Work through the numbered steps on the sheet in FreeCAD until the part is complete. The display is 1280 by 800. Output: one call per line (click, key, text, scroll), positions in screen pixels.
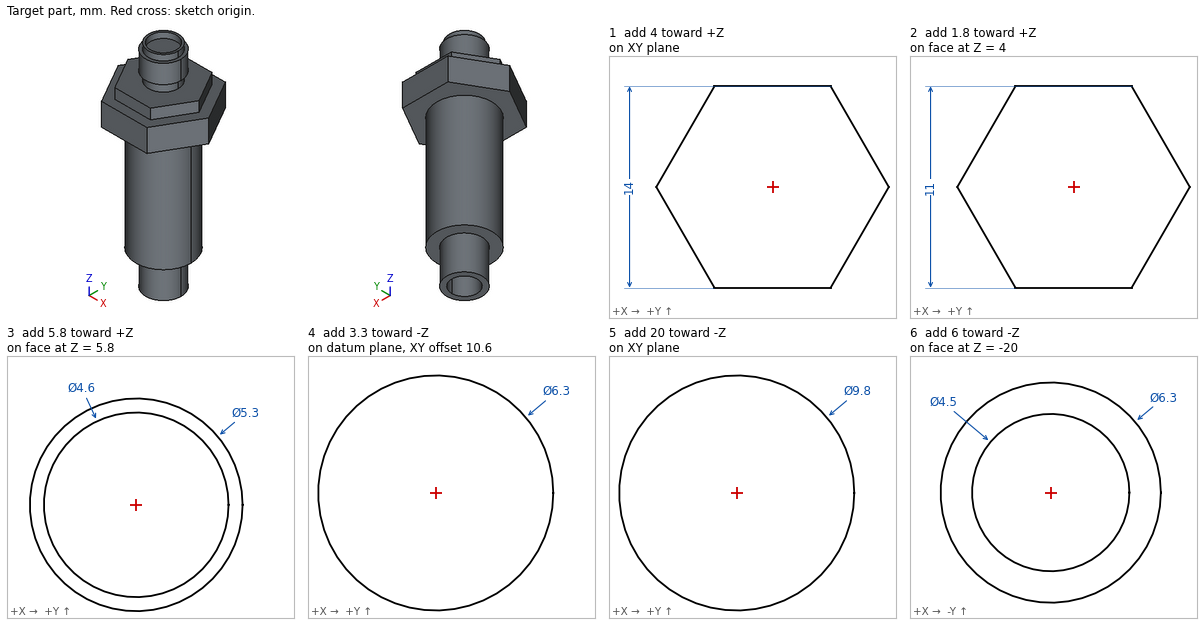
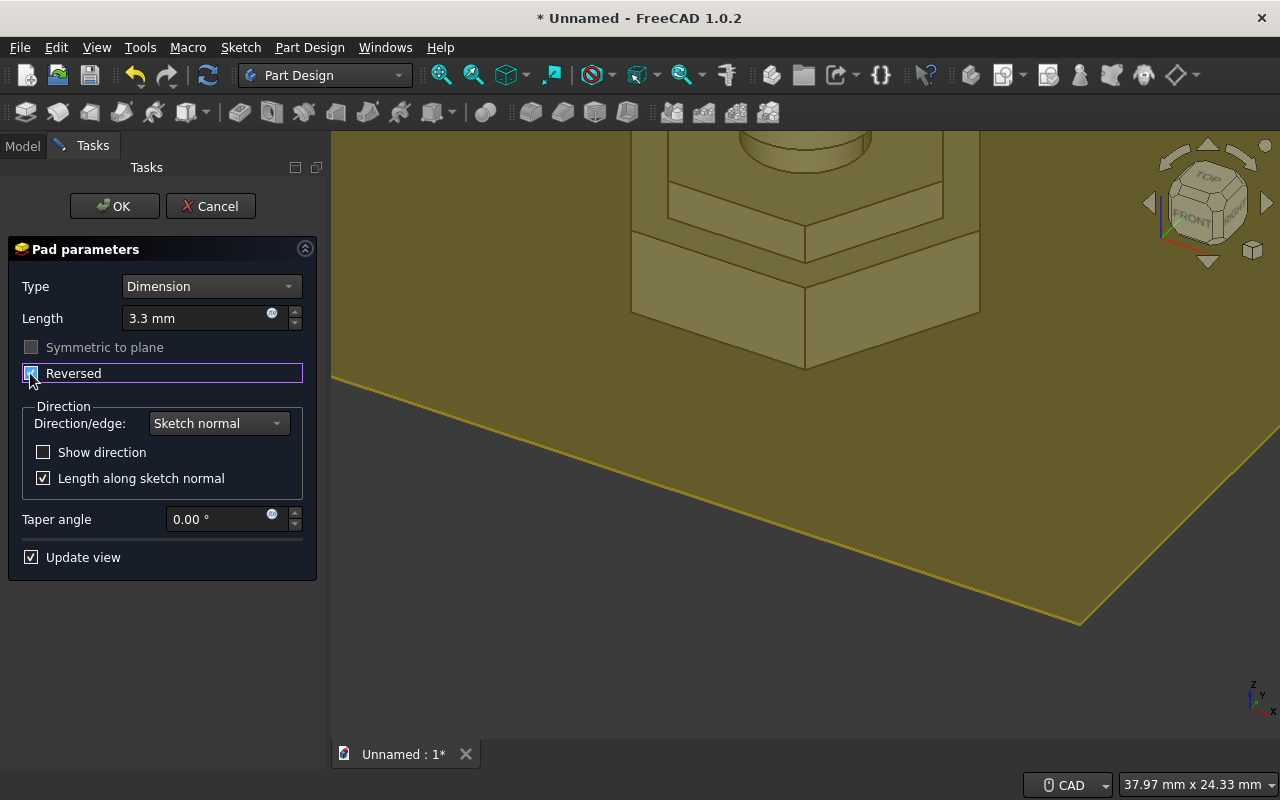
click(115, 206)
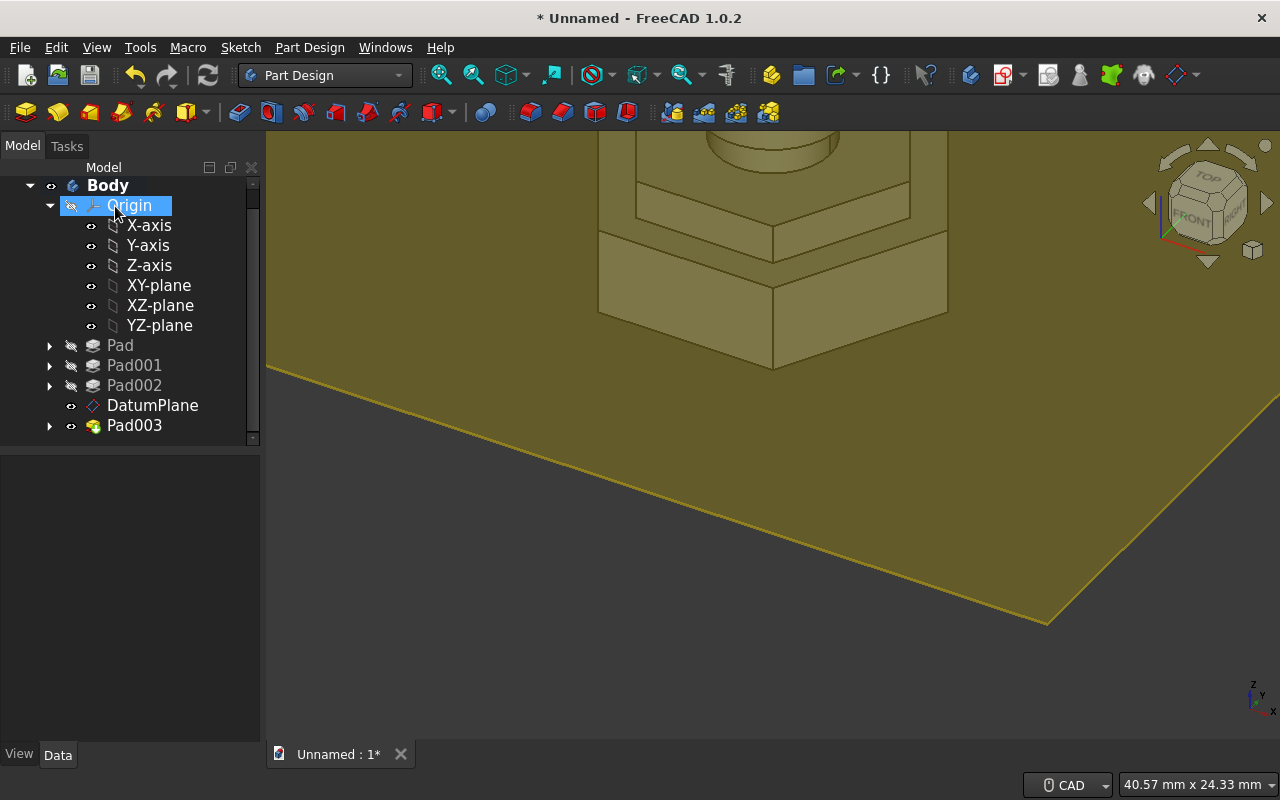
click(116, 406)
key(space)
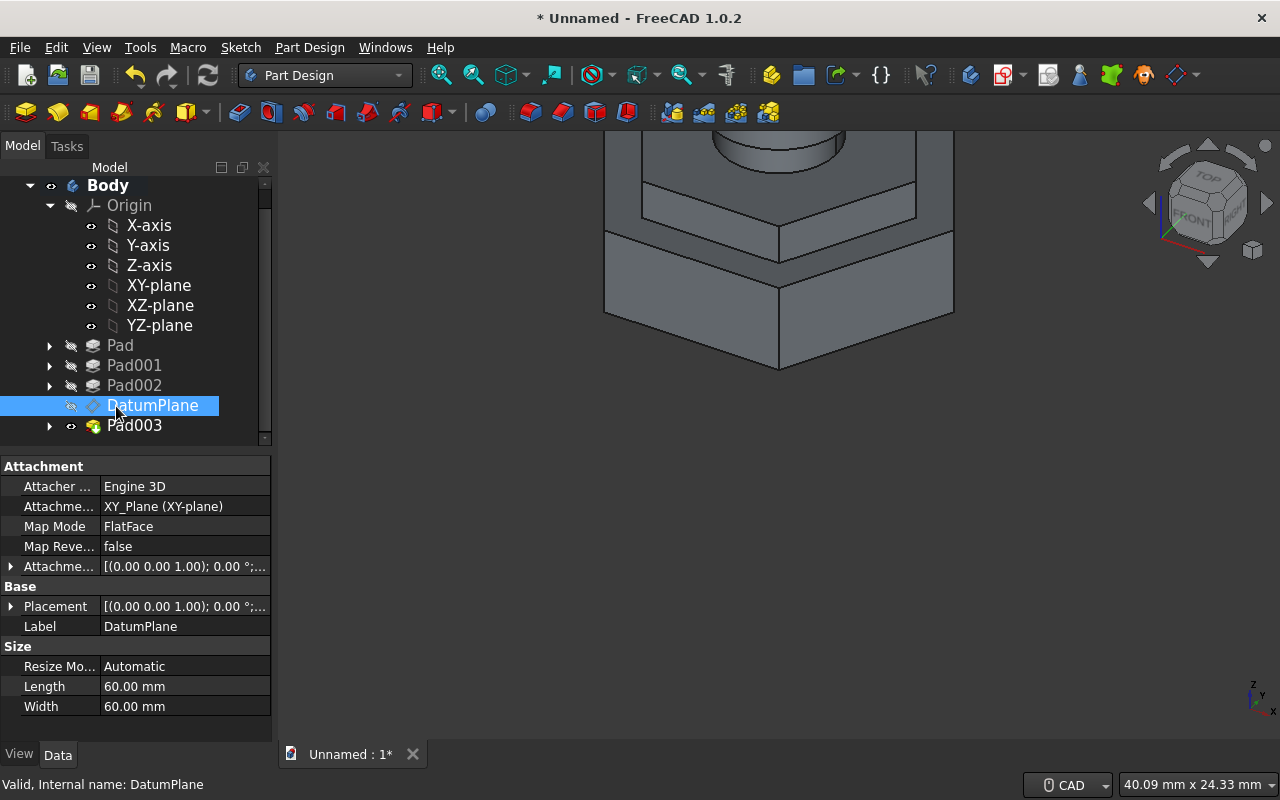
click(442, 76)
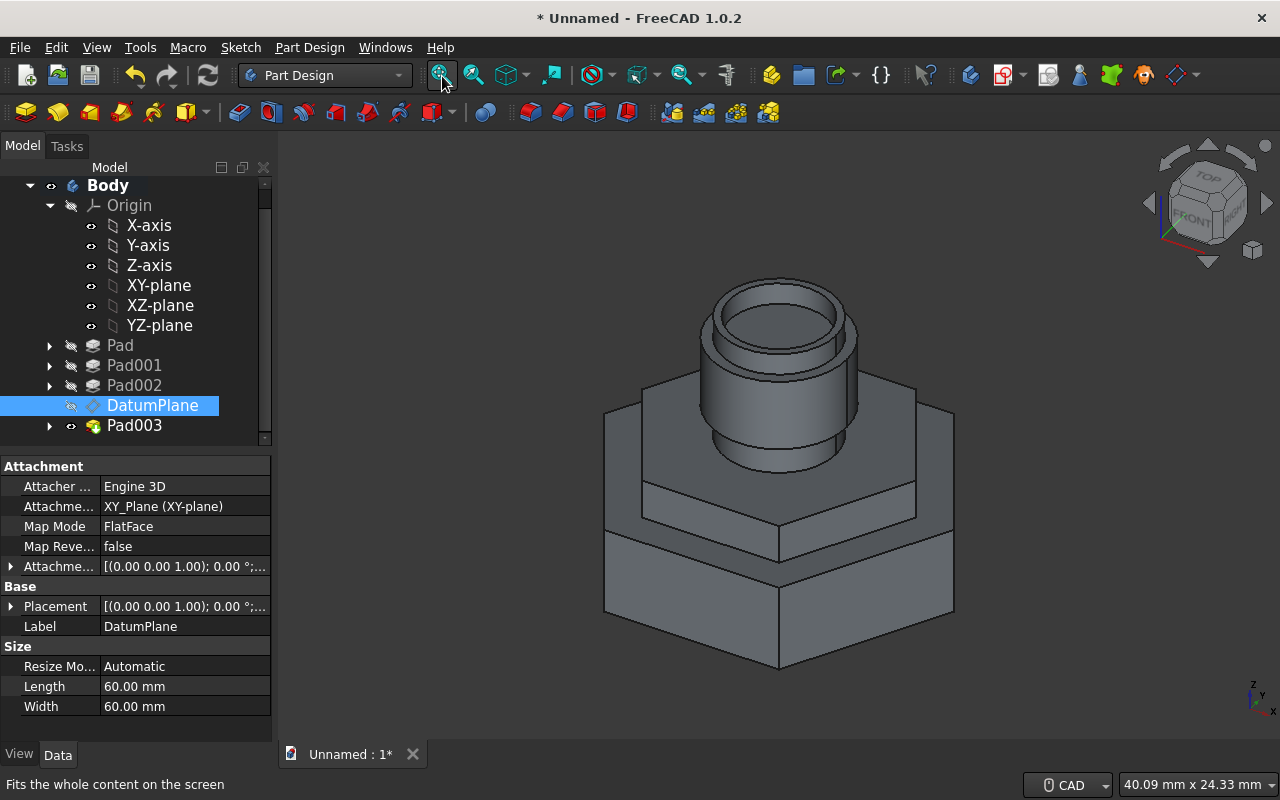
click(318, 699)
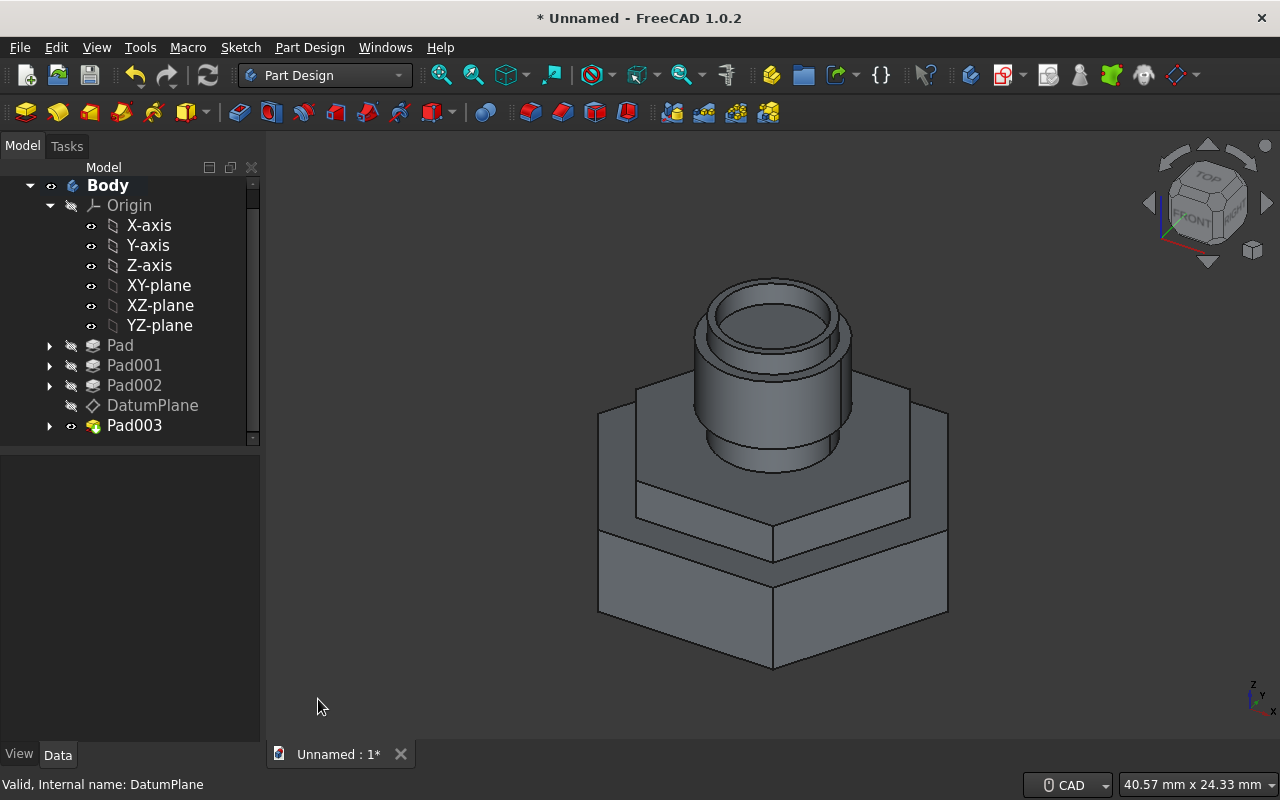
click(1004, 76)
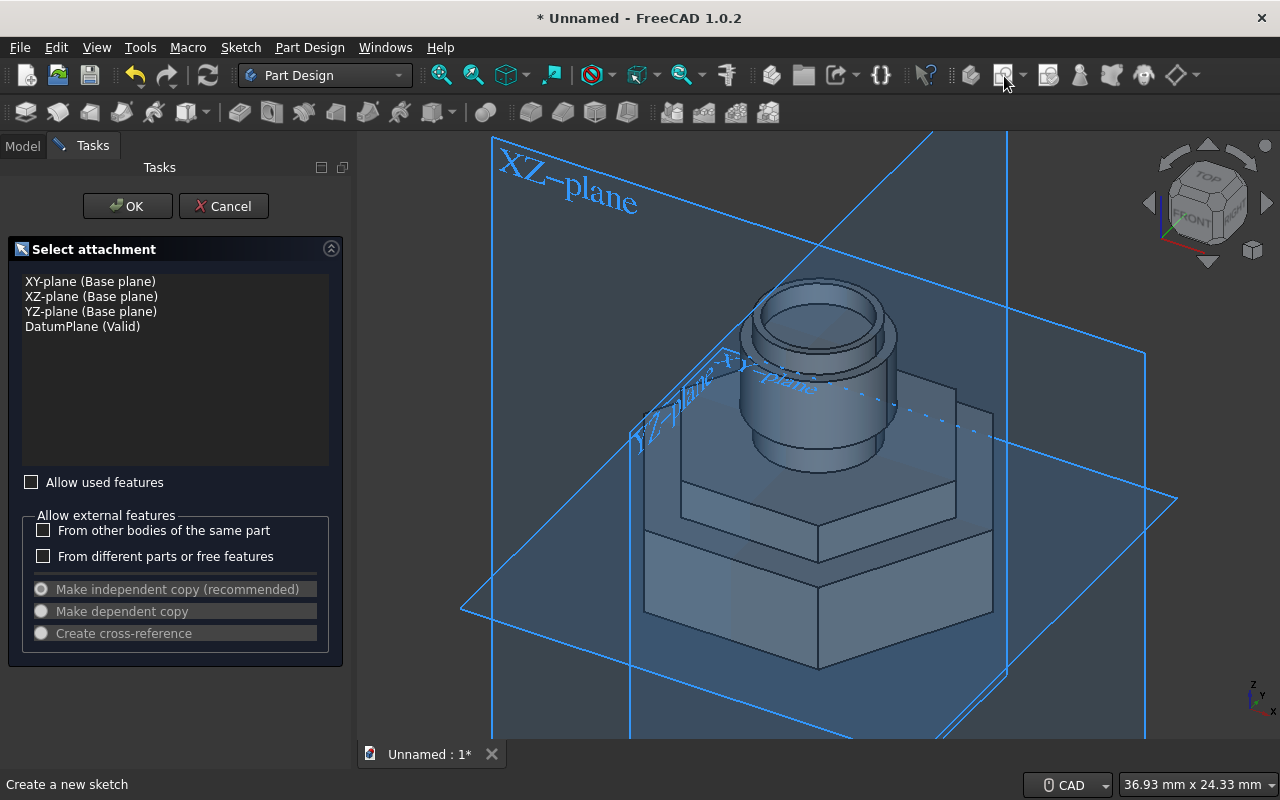
click(82, 282)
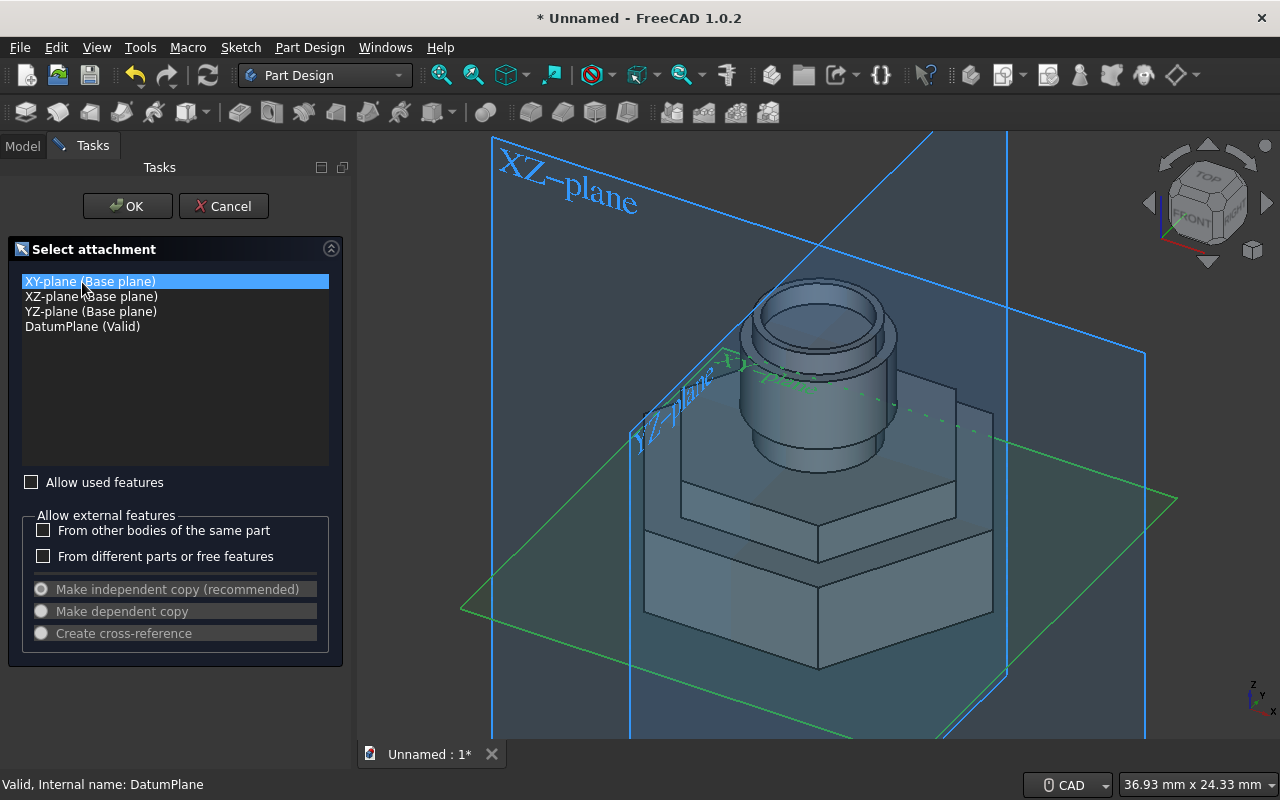
click(128, 206)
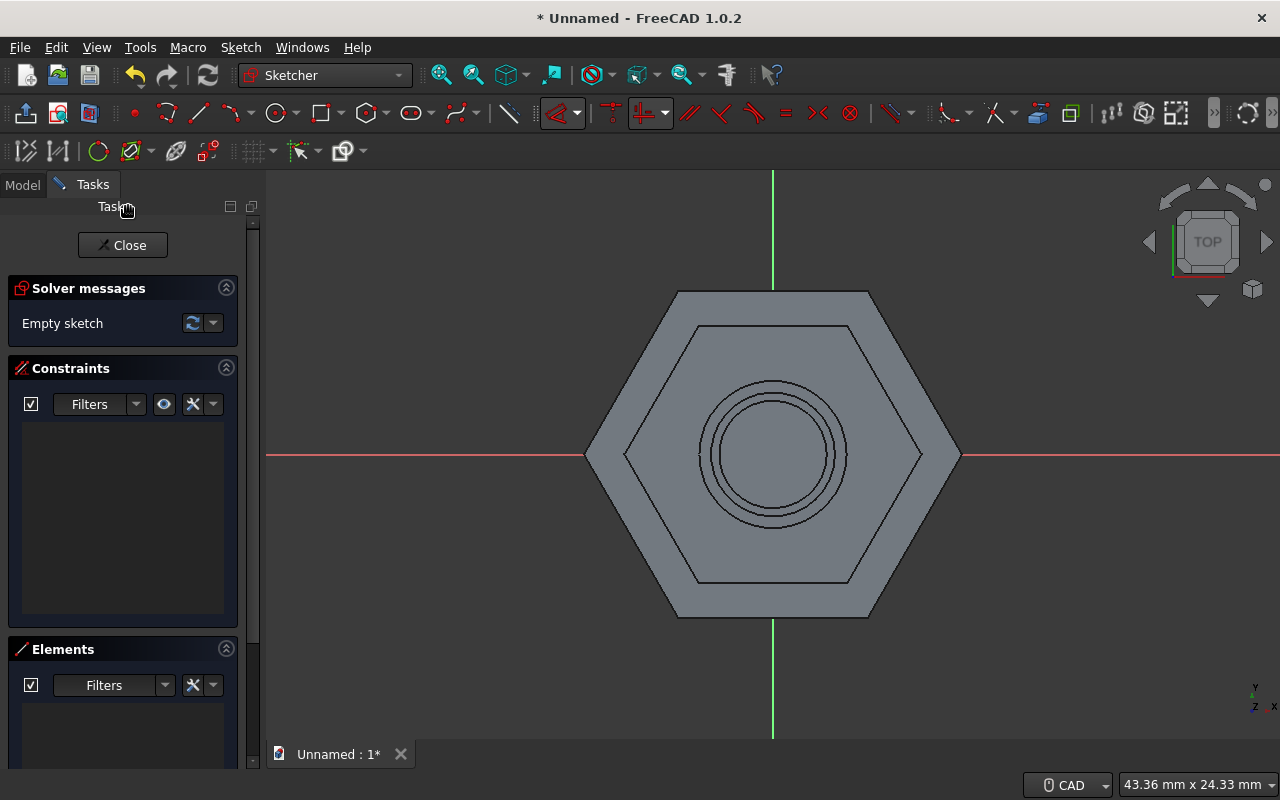
click(90, 114)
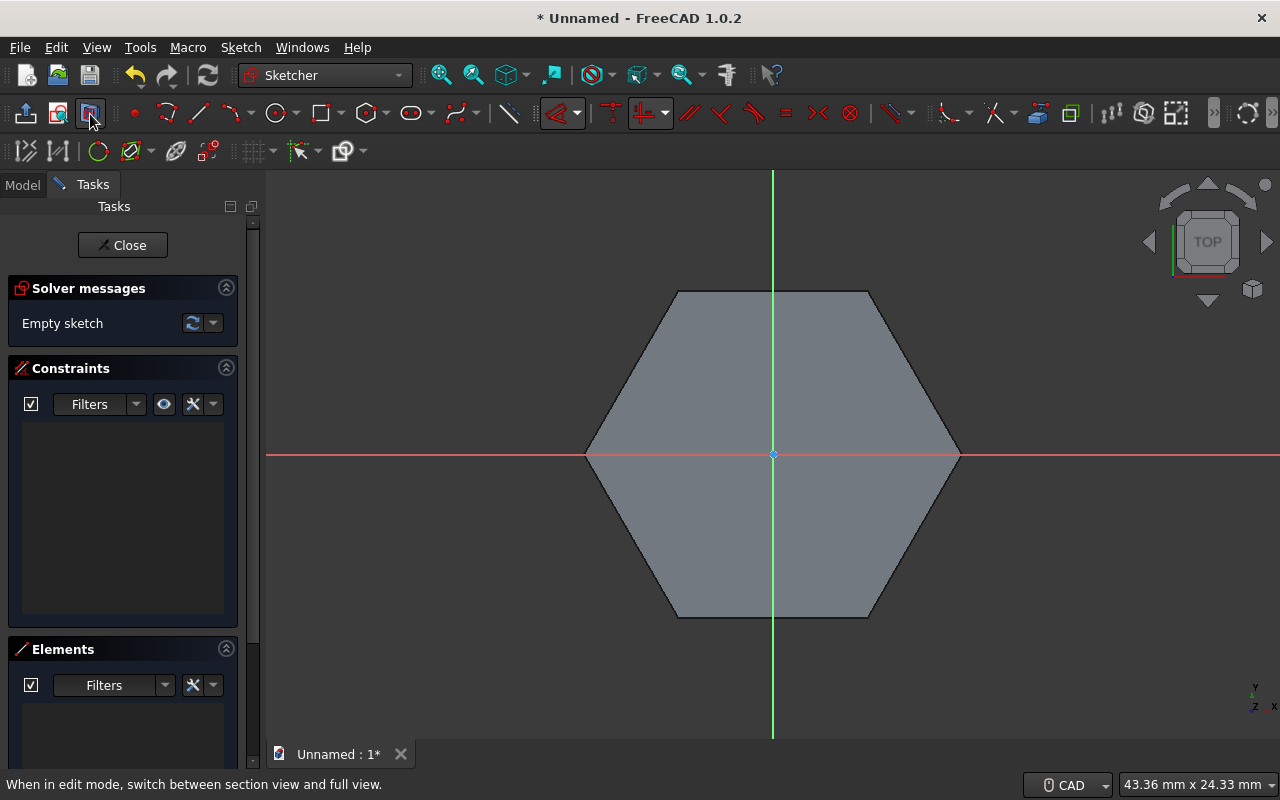
scroll(912, 455, up, 2)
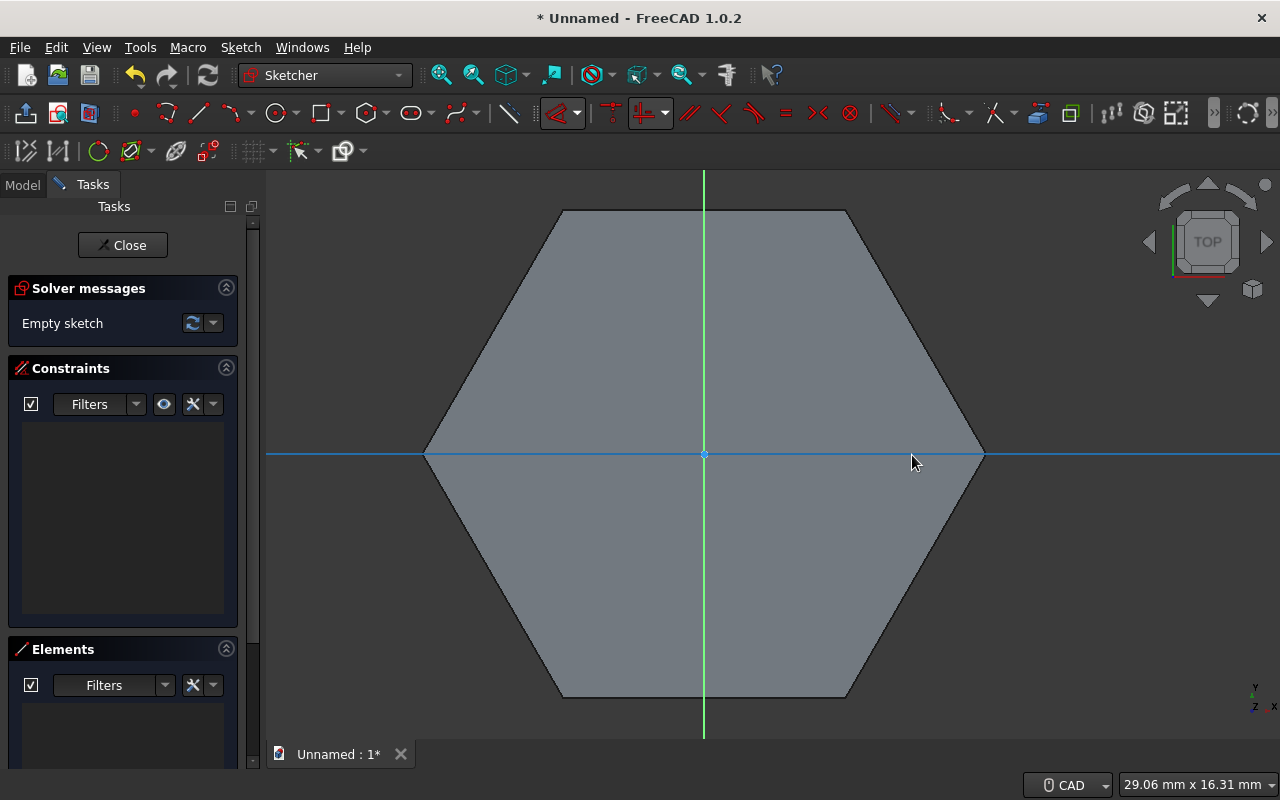
click(276, 114)